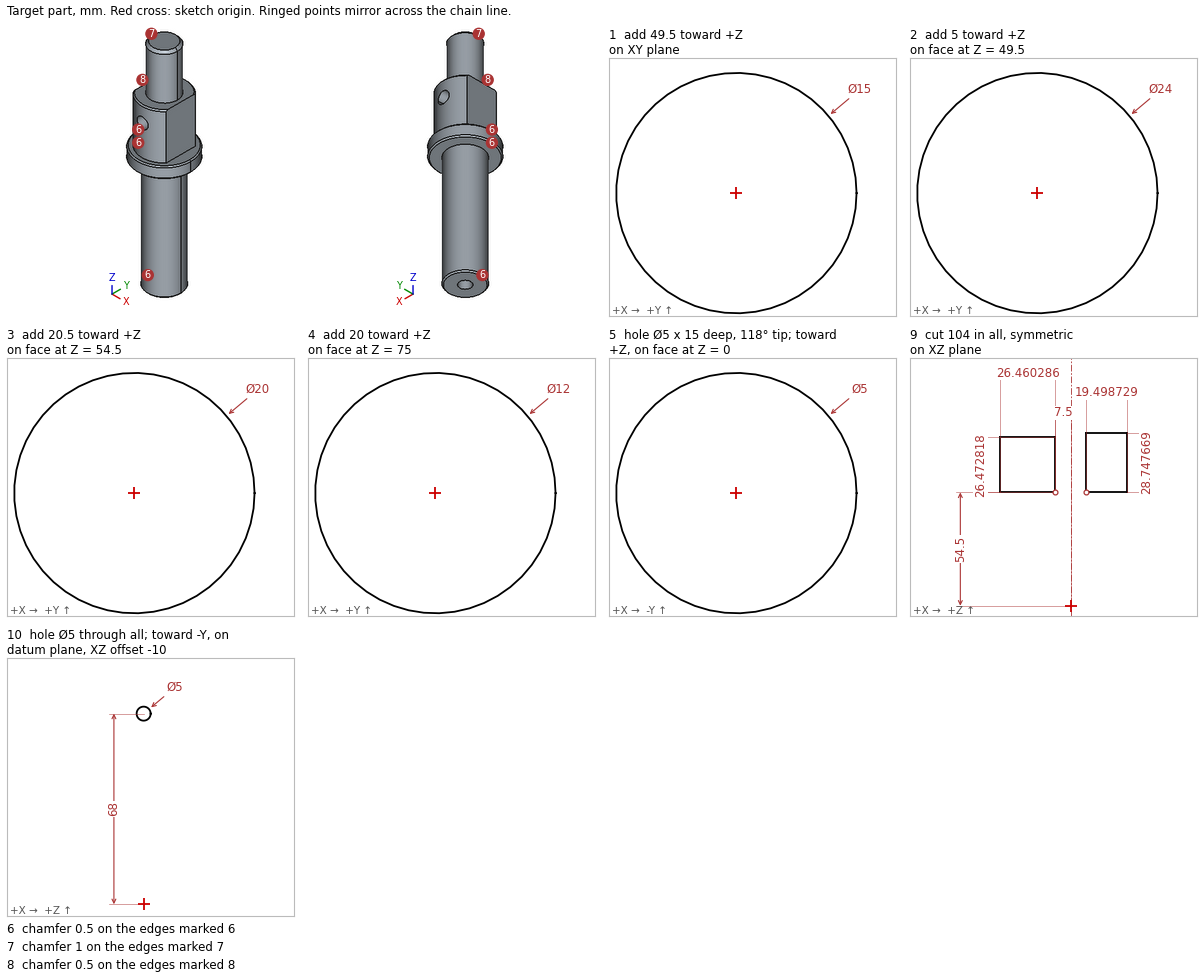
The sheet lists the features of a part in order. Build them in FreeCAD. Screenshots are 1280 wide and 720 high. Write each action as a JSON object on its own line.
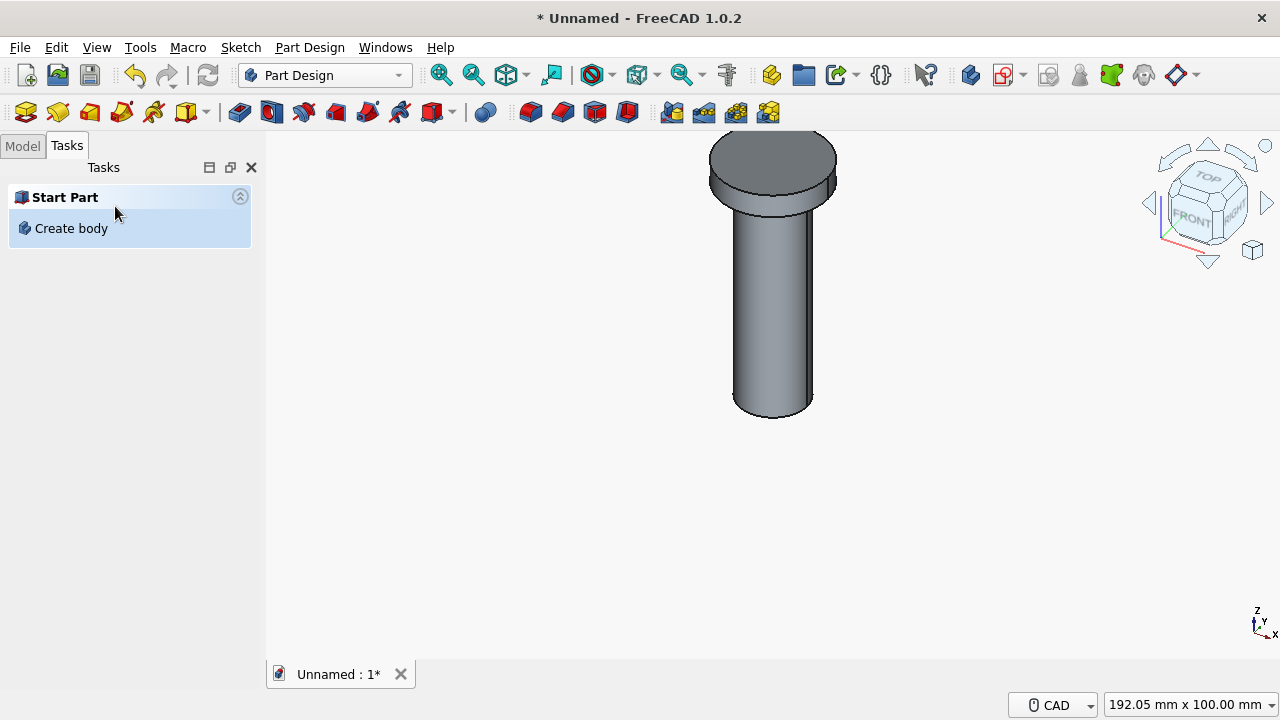
{"action": "key", "text": "v f"}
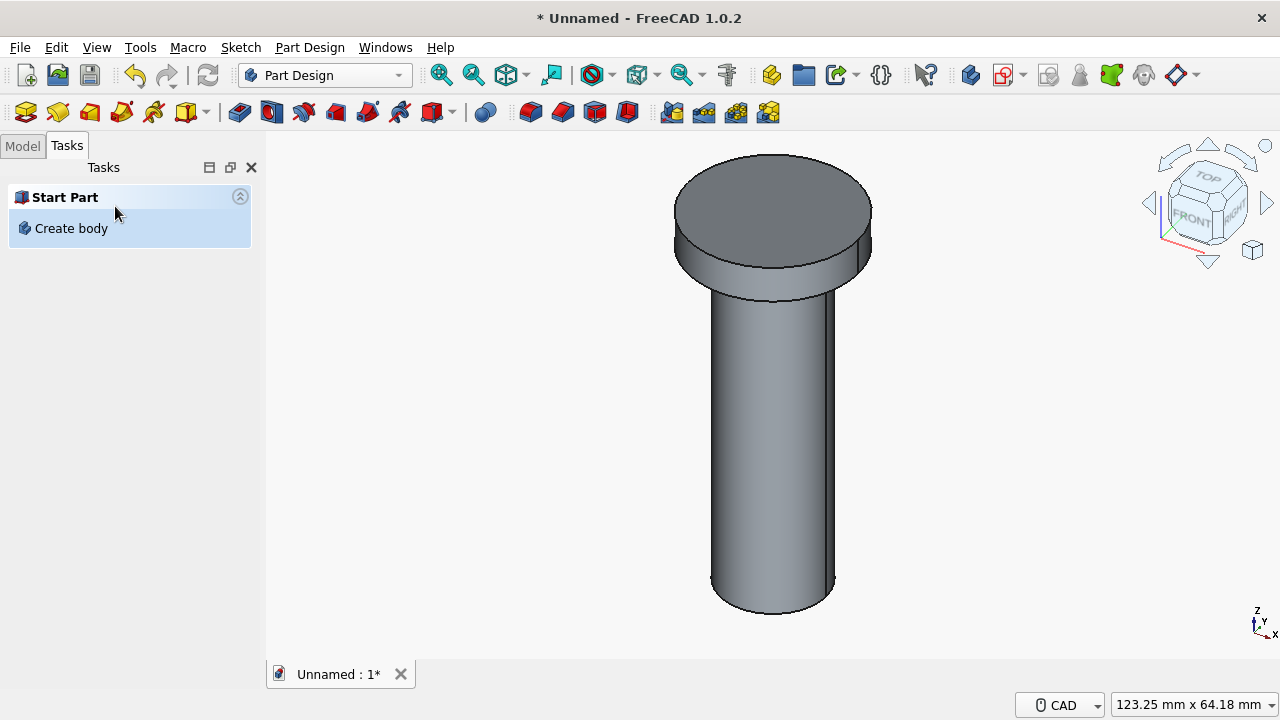
{"action": "left_click", "coordinate": [773, 210]}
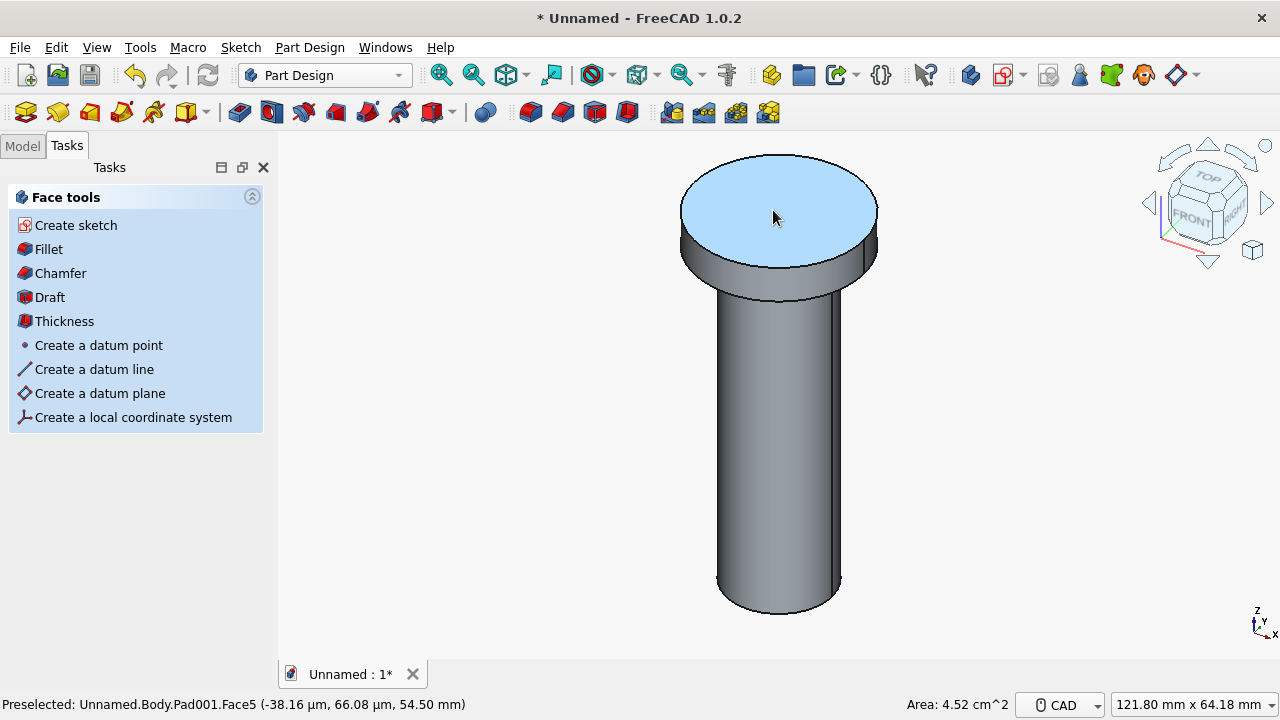
{"action": "left_click", "coordinate": [1004, 76]}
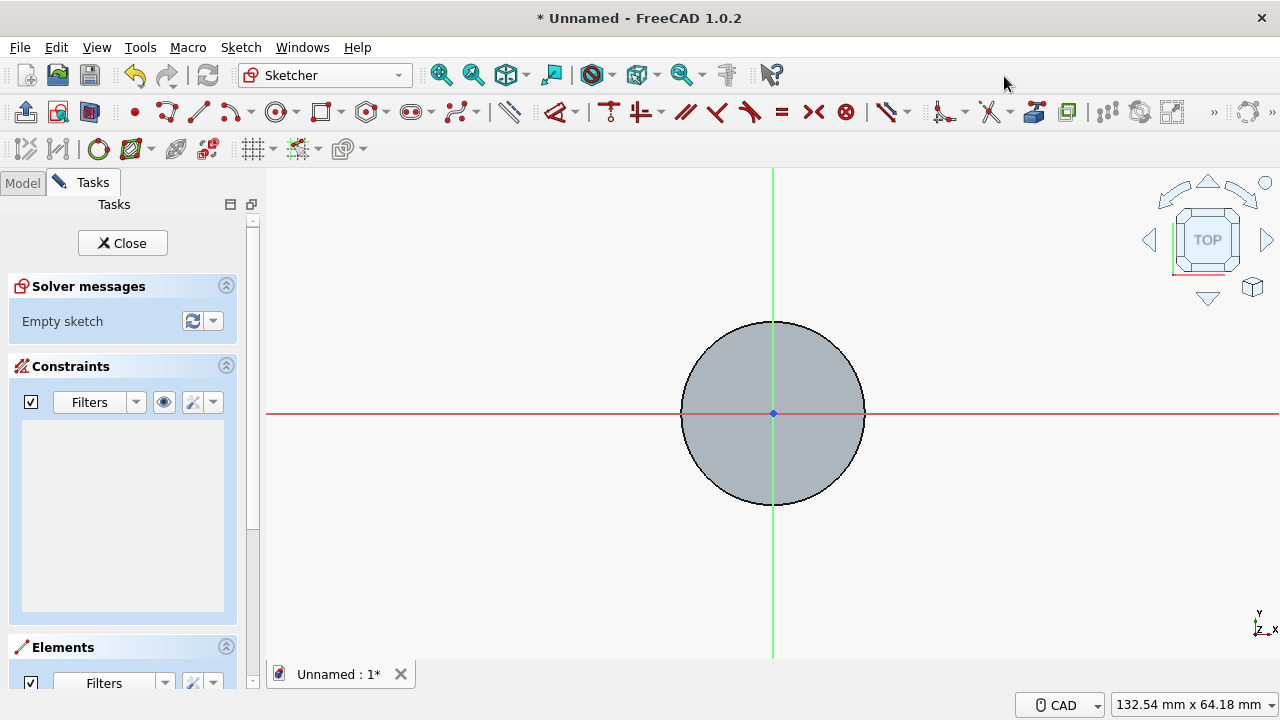
{"action": "scroll", "coordinate": [856, 414], "scroll_direction": "up", "scroll_amount": 3}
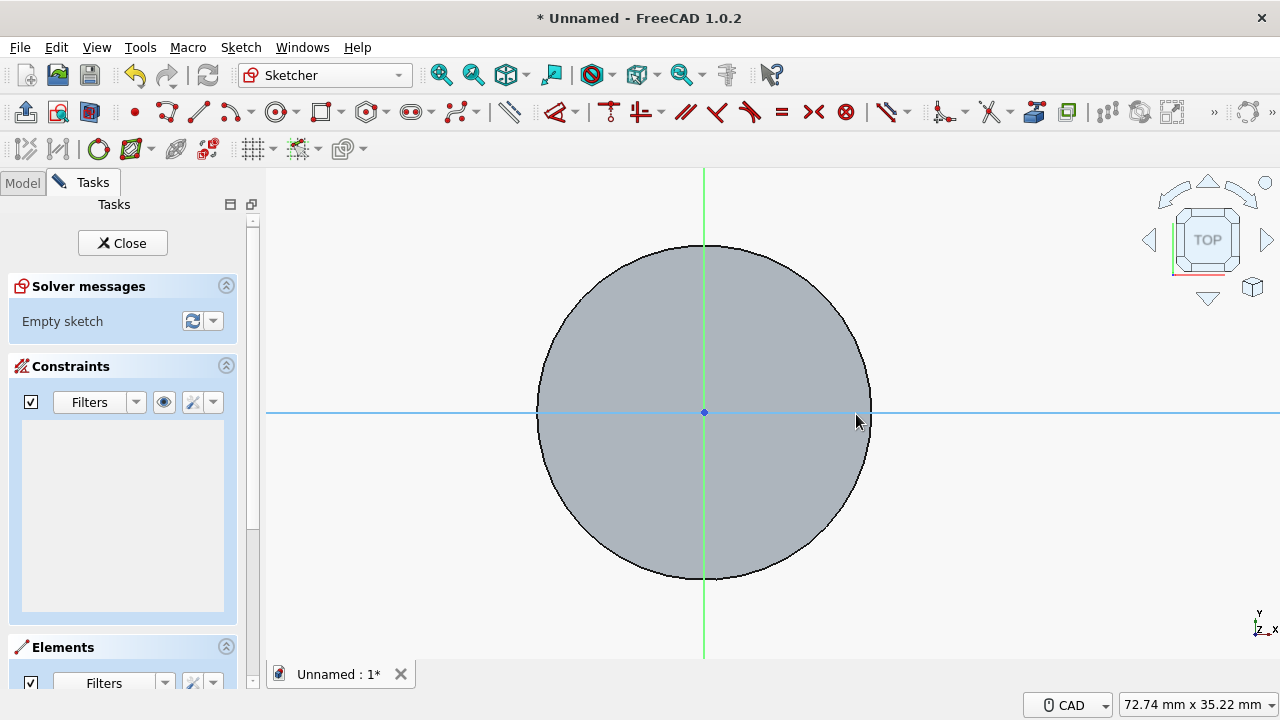
{"action": "key", "text": "g c"}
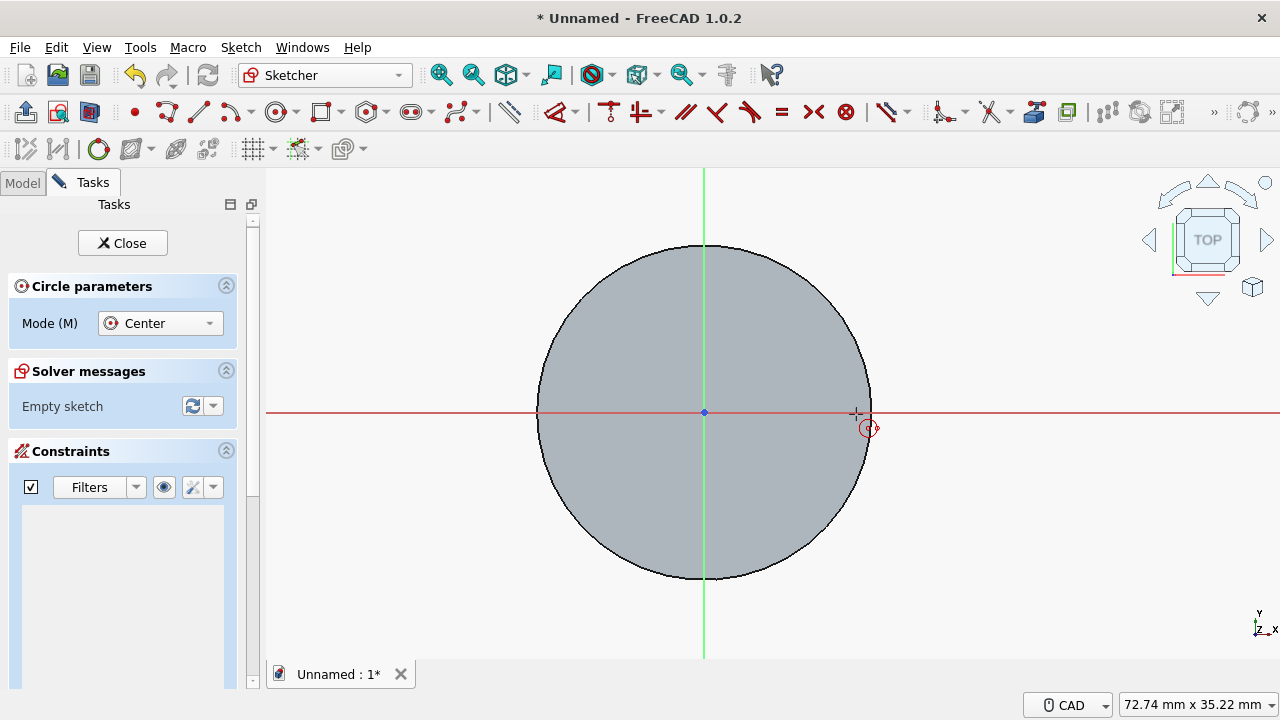
{"action": "left_click", "coordinate": [704, 413]}
{"action": "mouse_move", "coordinate": [803, 314]}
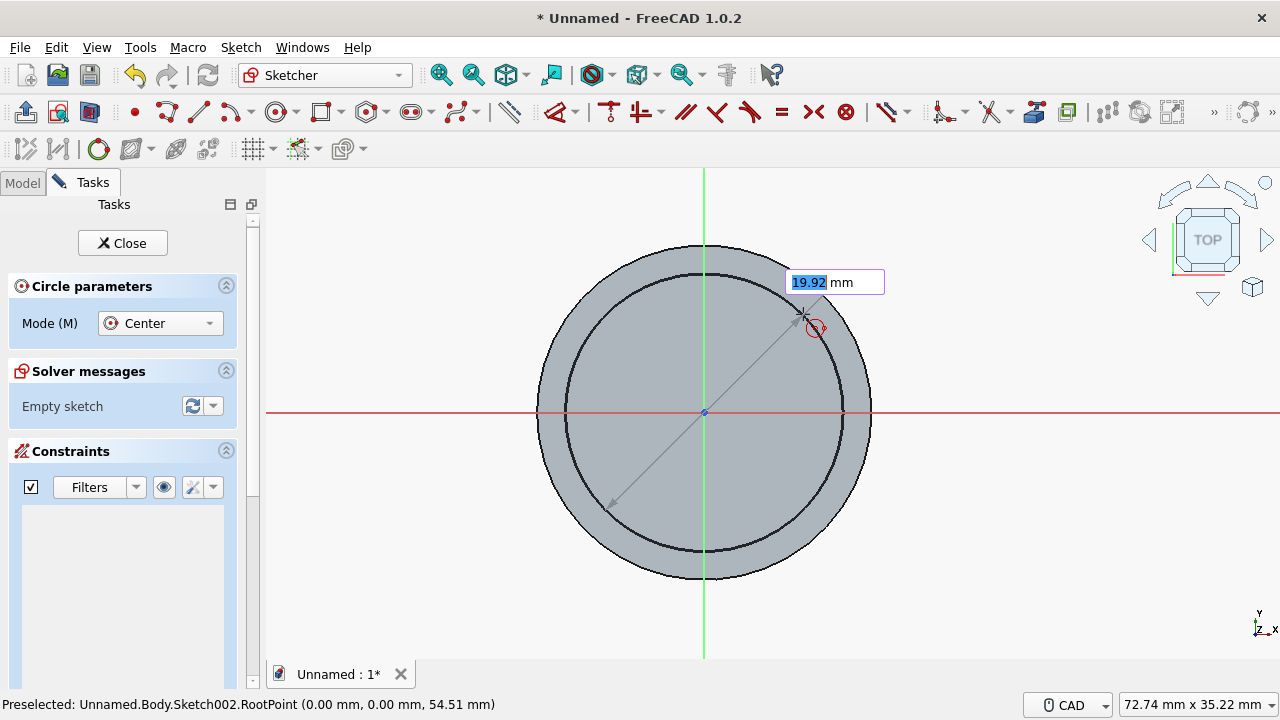
{"action": "type", "text": "20"}
{"action": "key", "text": "Return"}
{"action": "key", "text": "Escape"}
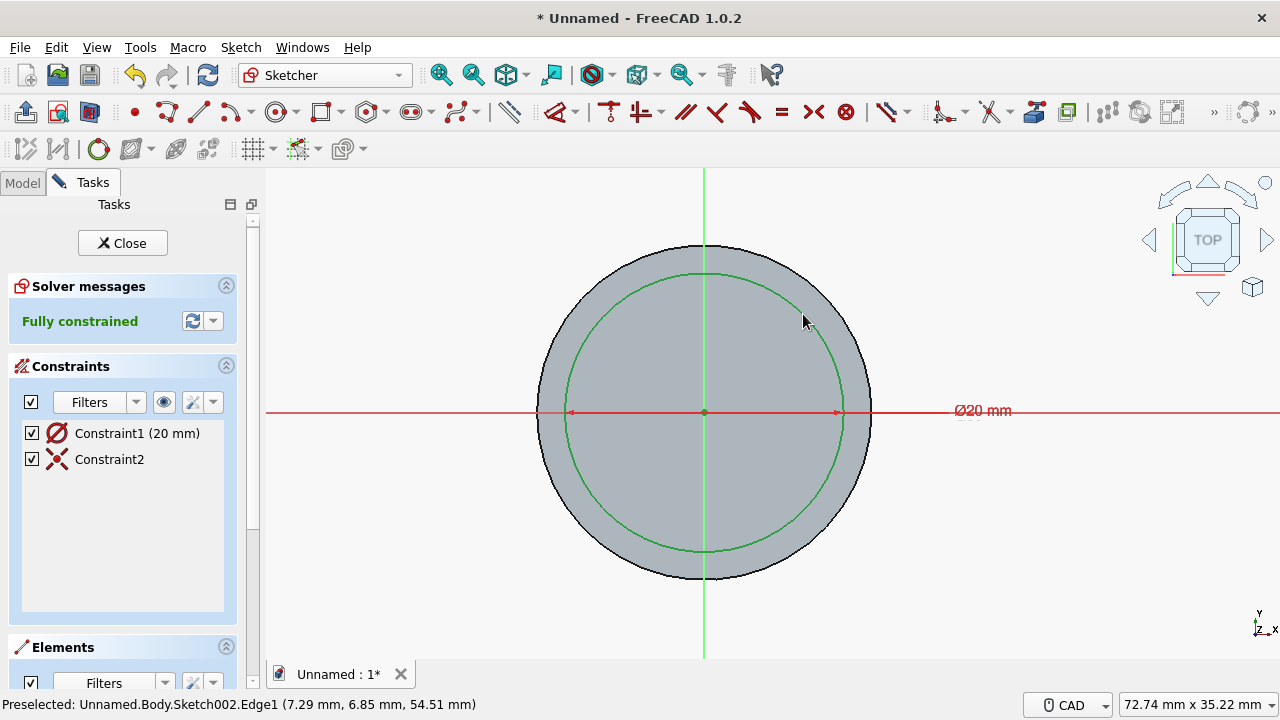
{"action": "left_click", "coordinate": [123, 243]}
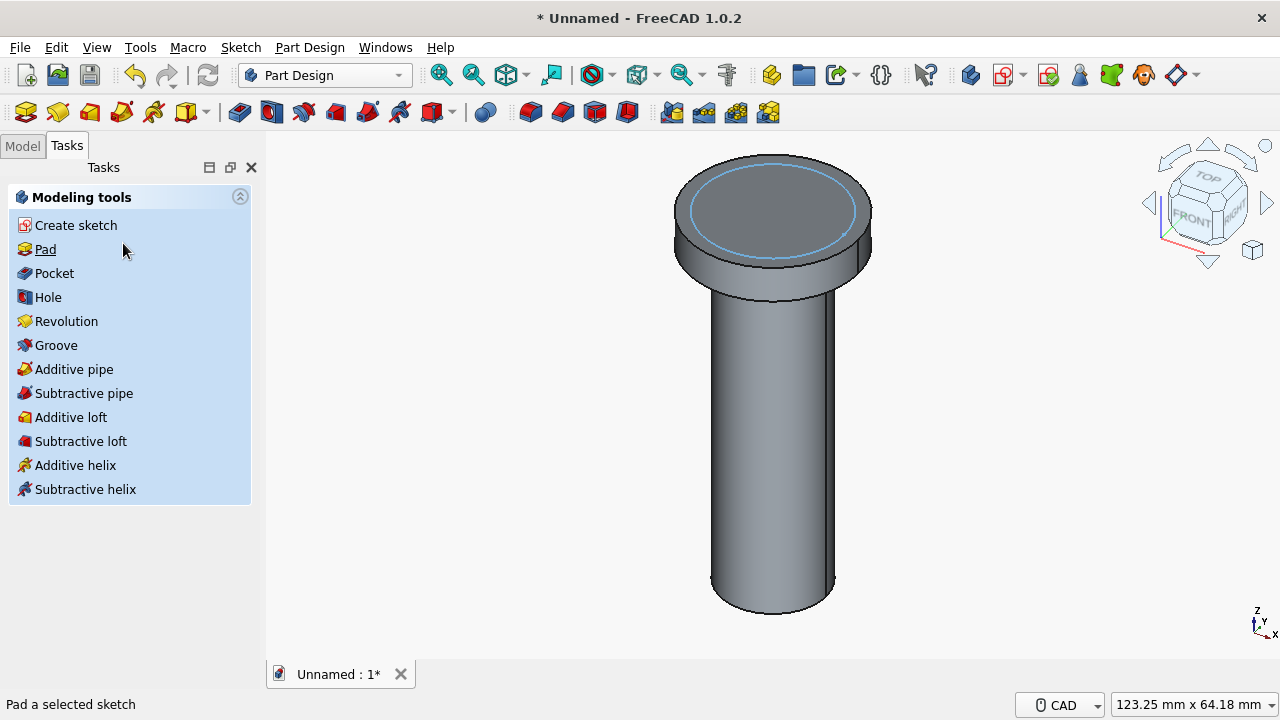
{"action": "left_click", "coordinate": [26, 112]}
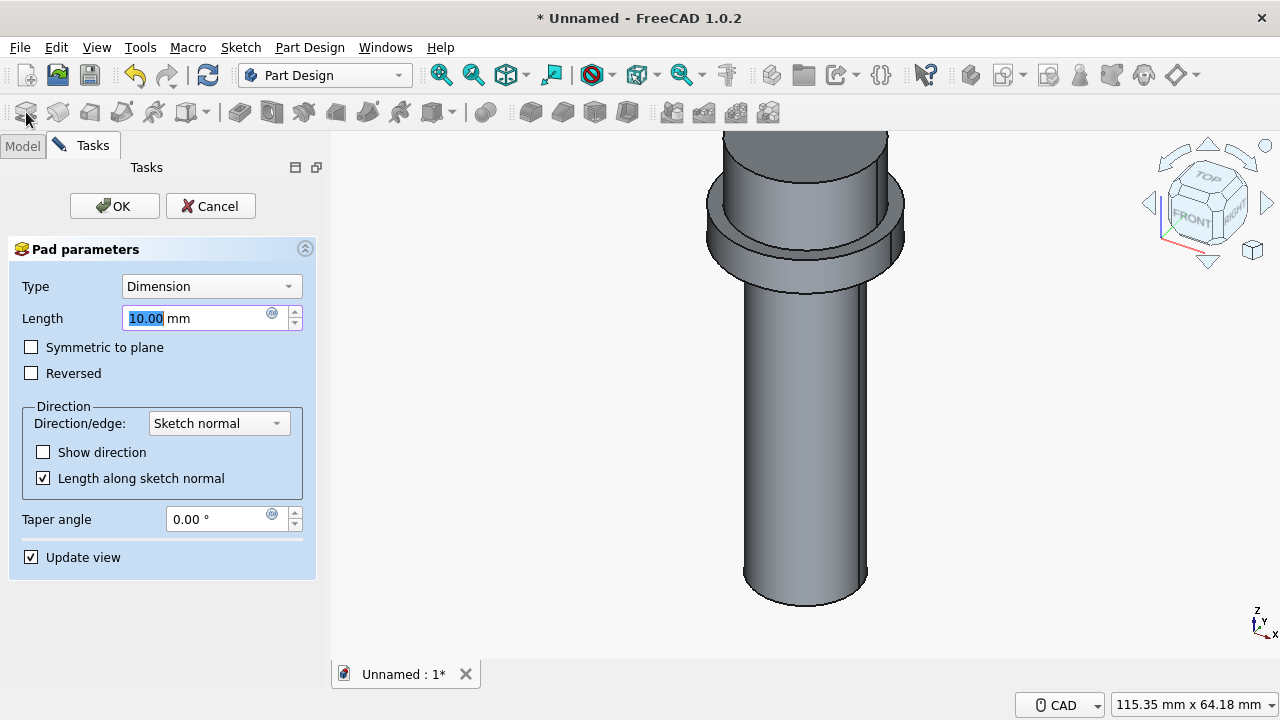
{"action": "type", "text": "20.5"}
{"action": "key", "text": "Tab"}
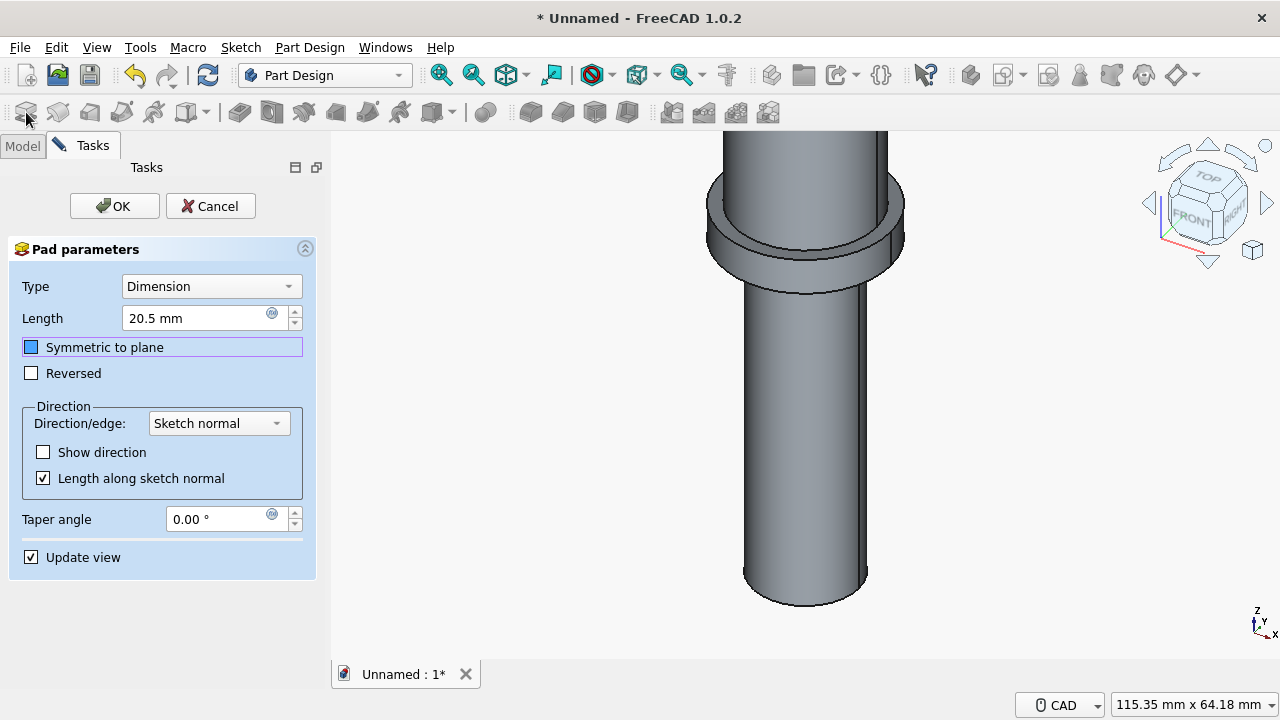
{"action": "left_click", "coordinate": [115, 206]}